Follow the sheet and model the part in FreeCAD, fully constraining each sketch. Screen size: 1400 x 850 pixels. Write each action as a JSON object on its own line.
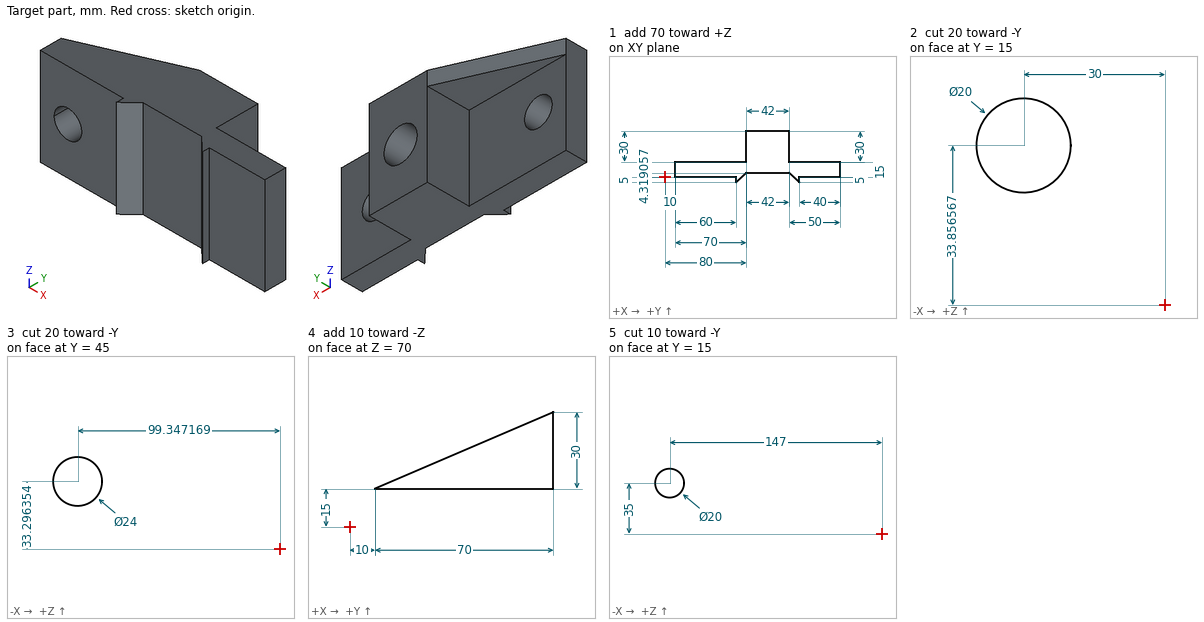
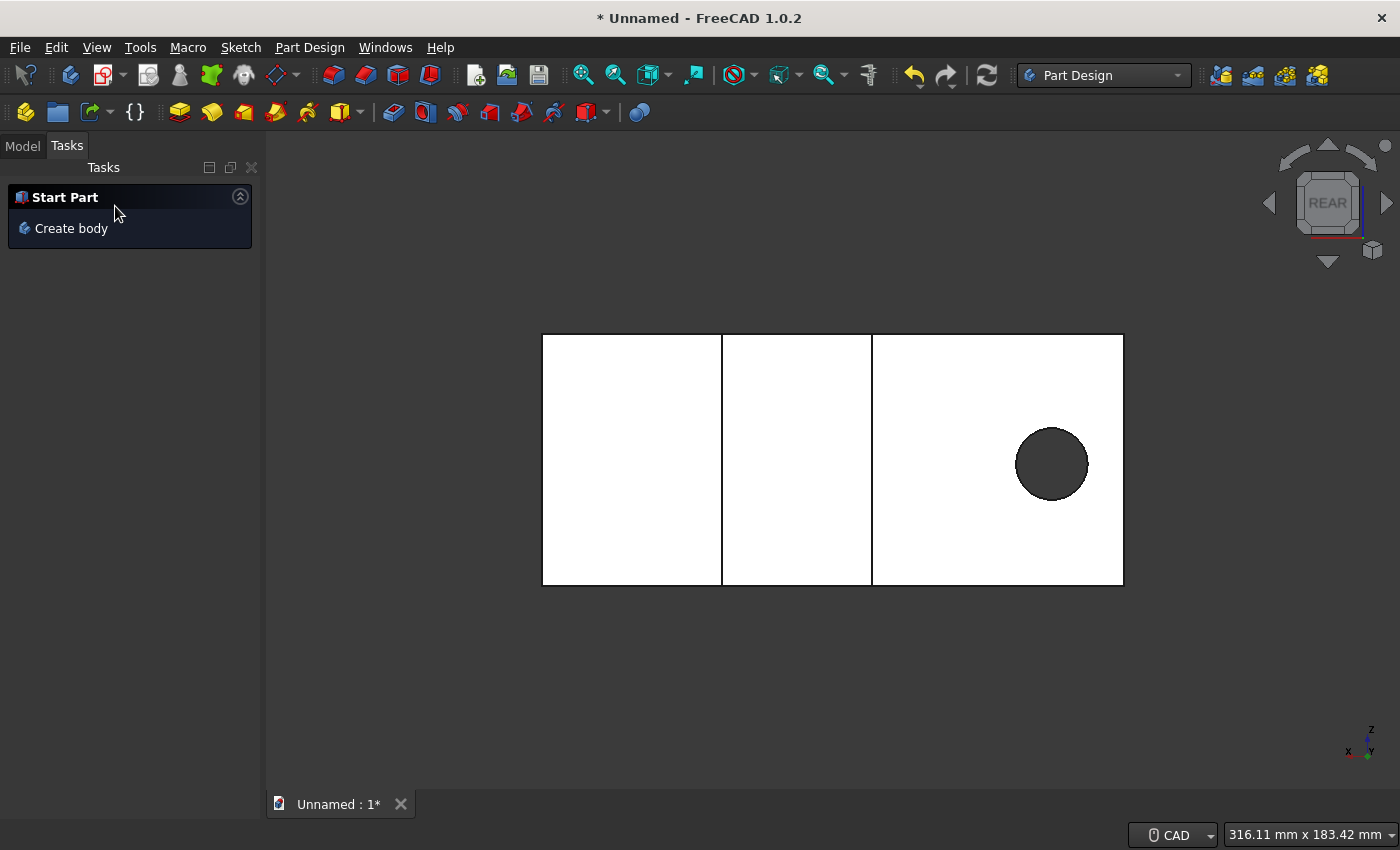
{"action": "left_click", "coordinate": [797, 423]}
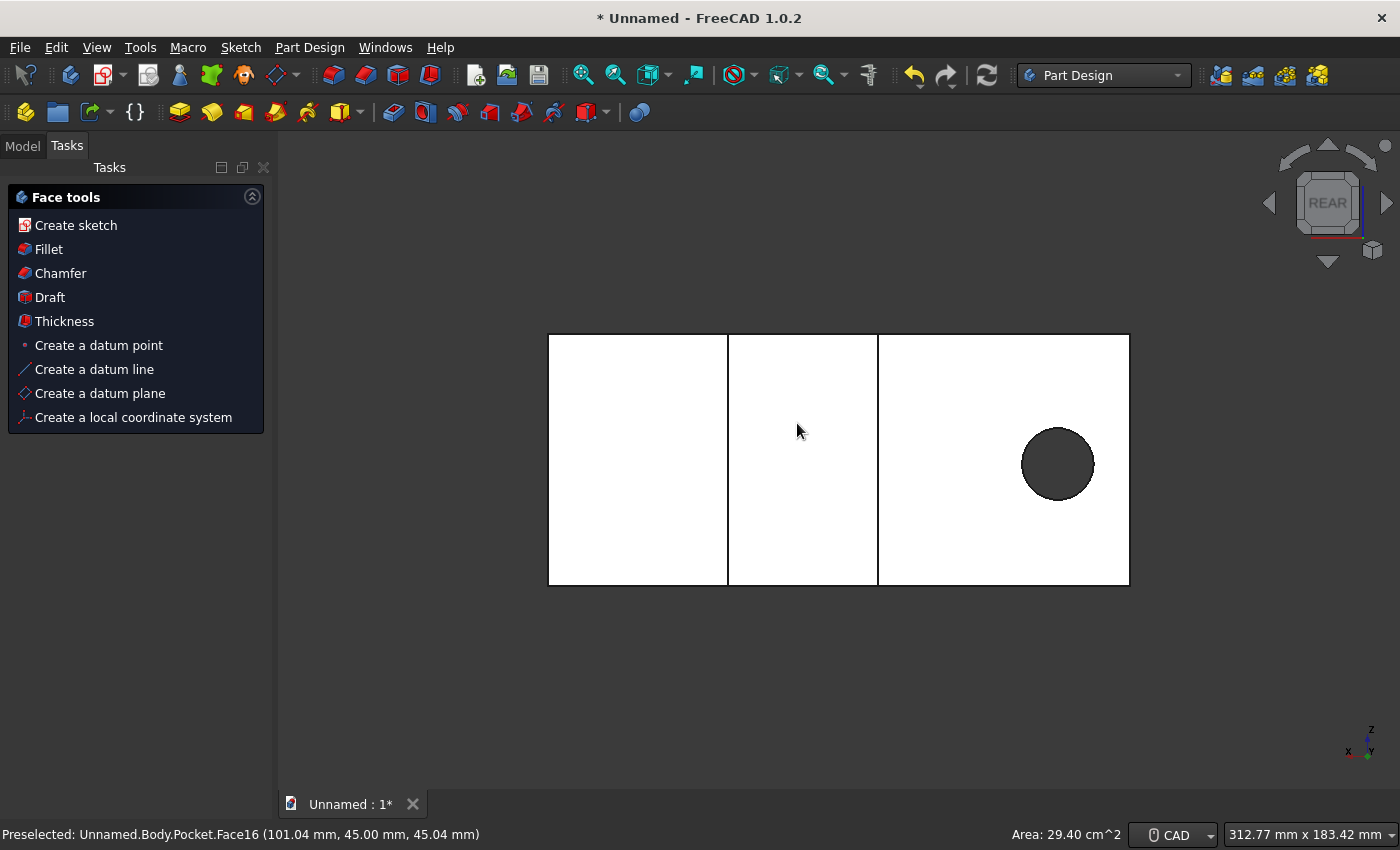
{"action": "left_click", "coordinate": [104, 76]}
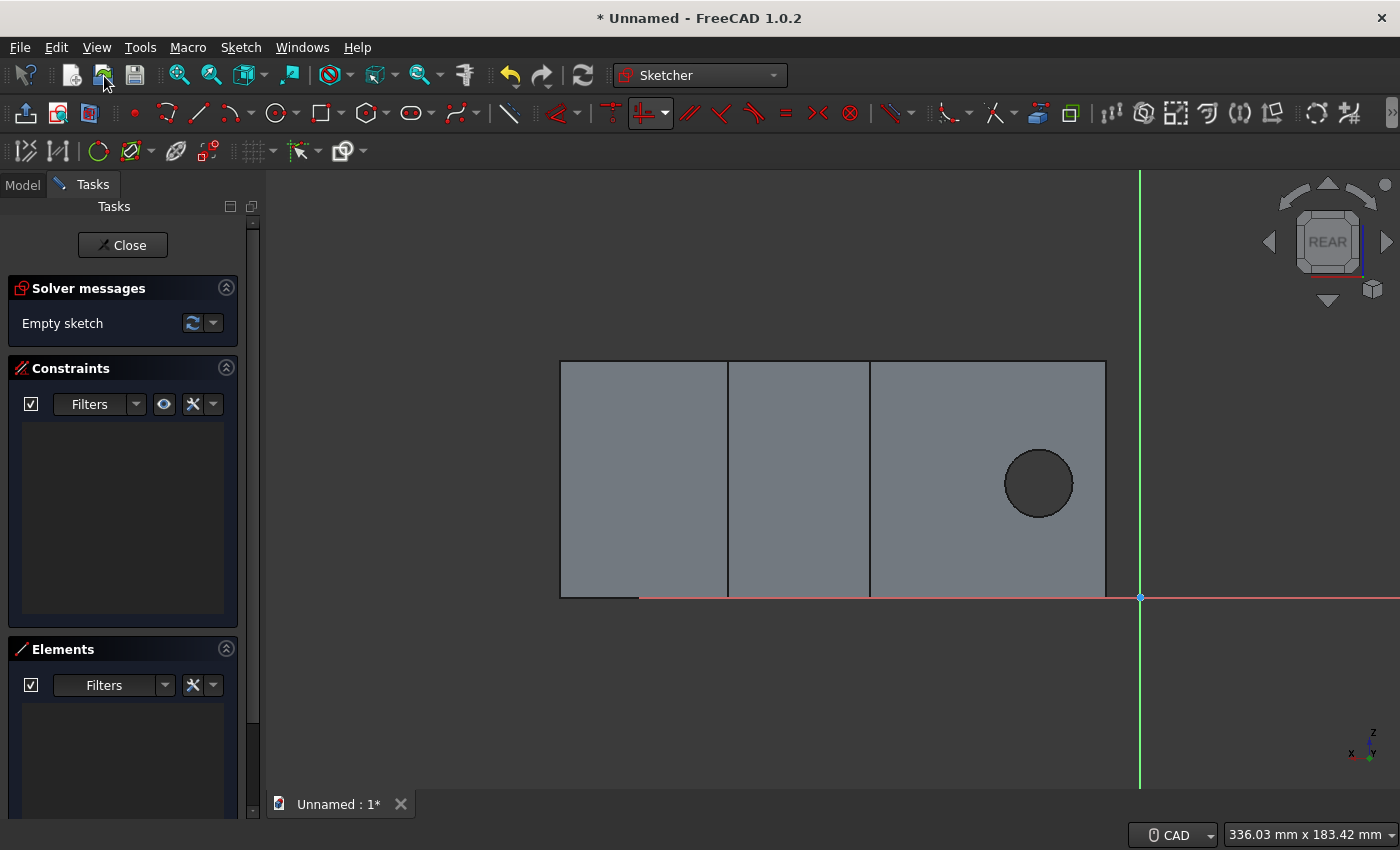
{"action": "scroll", "coordinate": [815, 487], "scroll_direction": "up", "scroll_amount": 8}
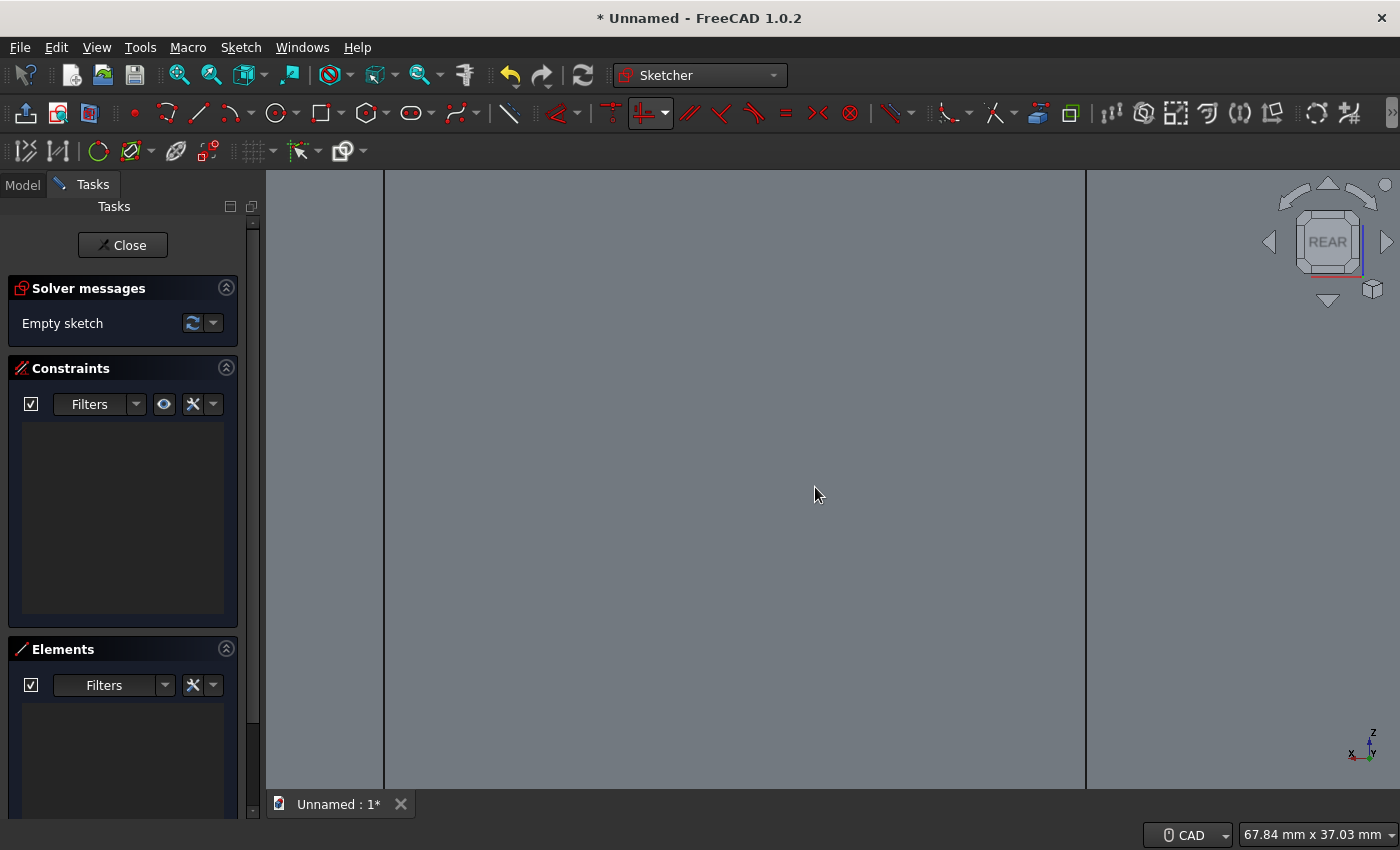
{"action": "left_click", "coordinate": [276, 114]}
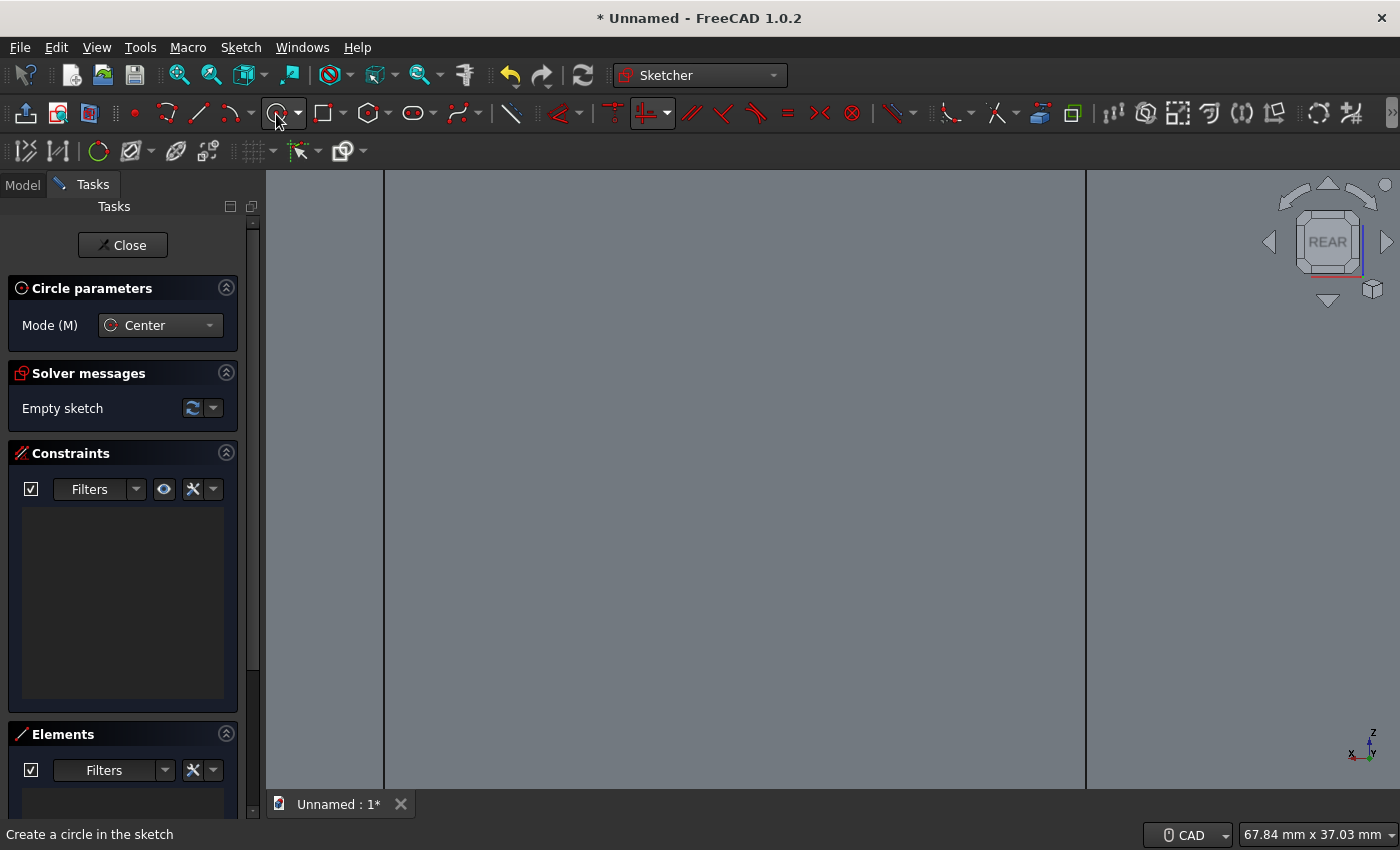
{"action": "left_click", "coordinate": [763, 476]}
{"action": "mouse_move", "coordinate": [905, 334]}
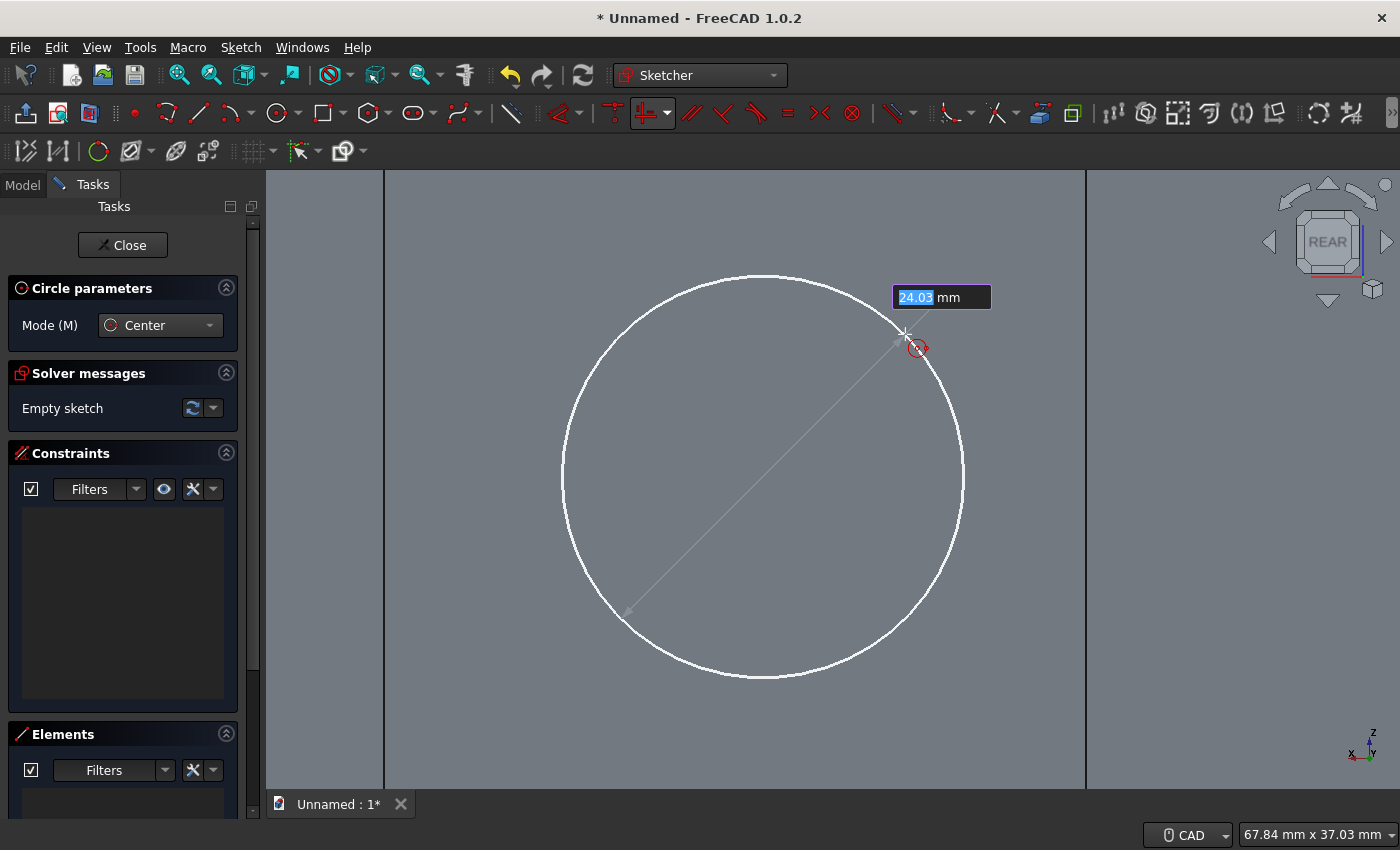
{"action": "type", "text": "24"}
{"action": "key", "text": "Return"}
{"action": "key", "text": "Escape"}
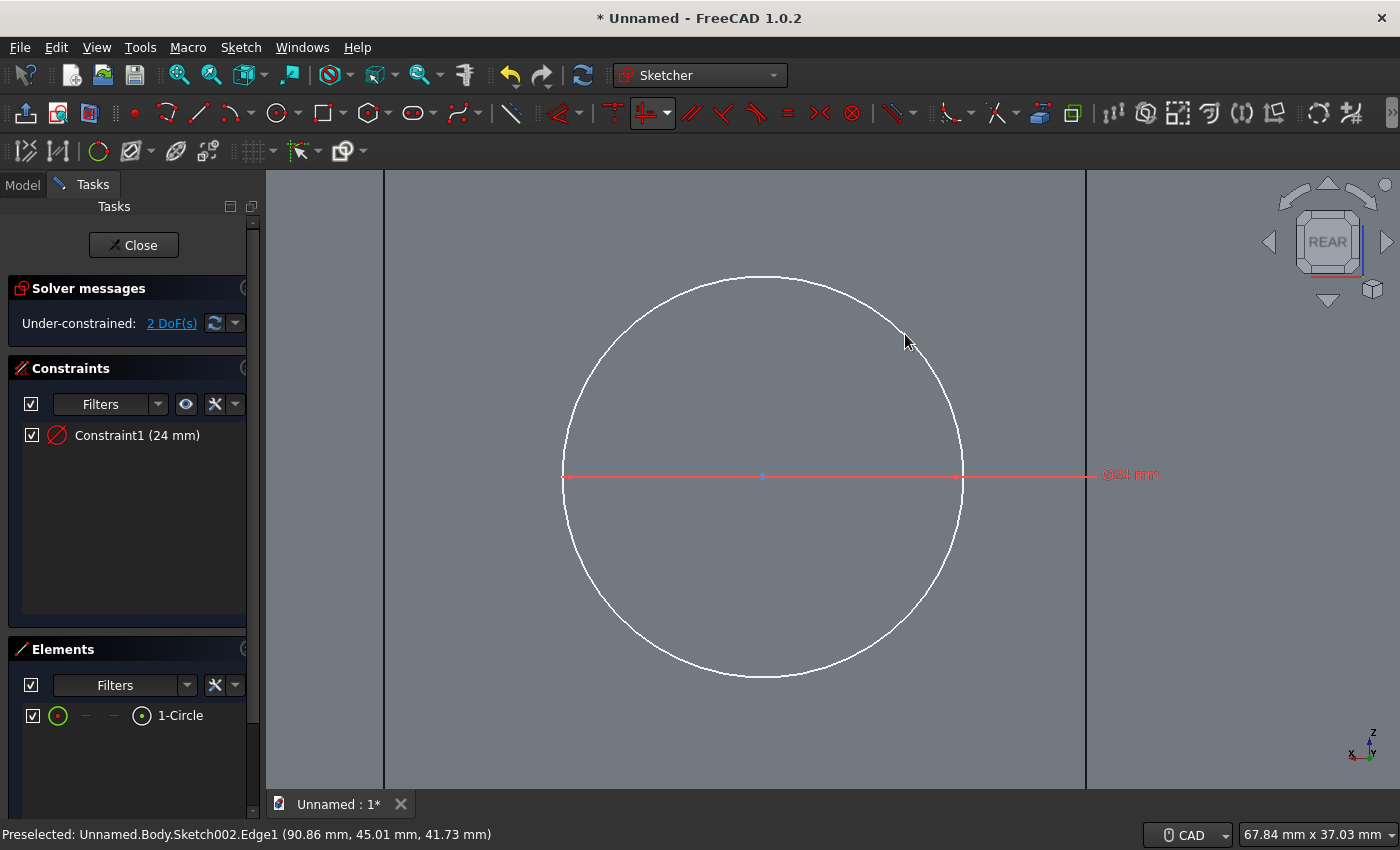
{"action": "left_click", "coordinate": [558, 114]}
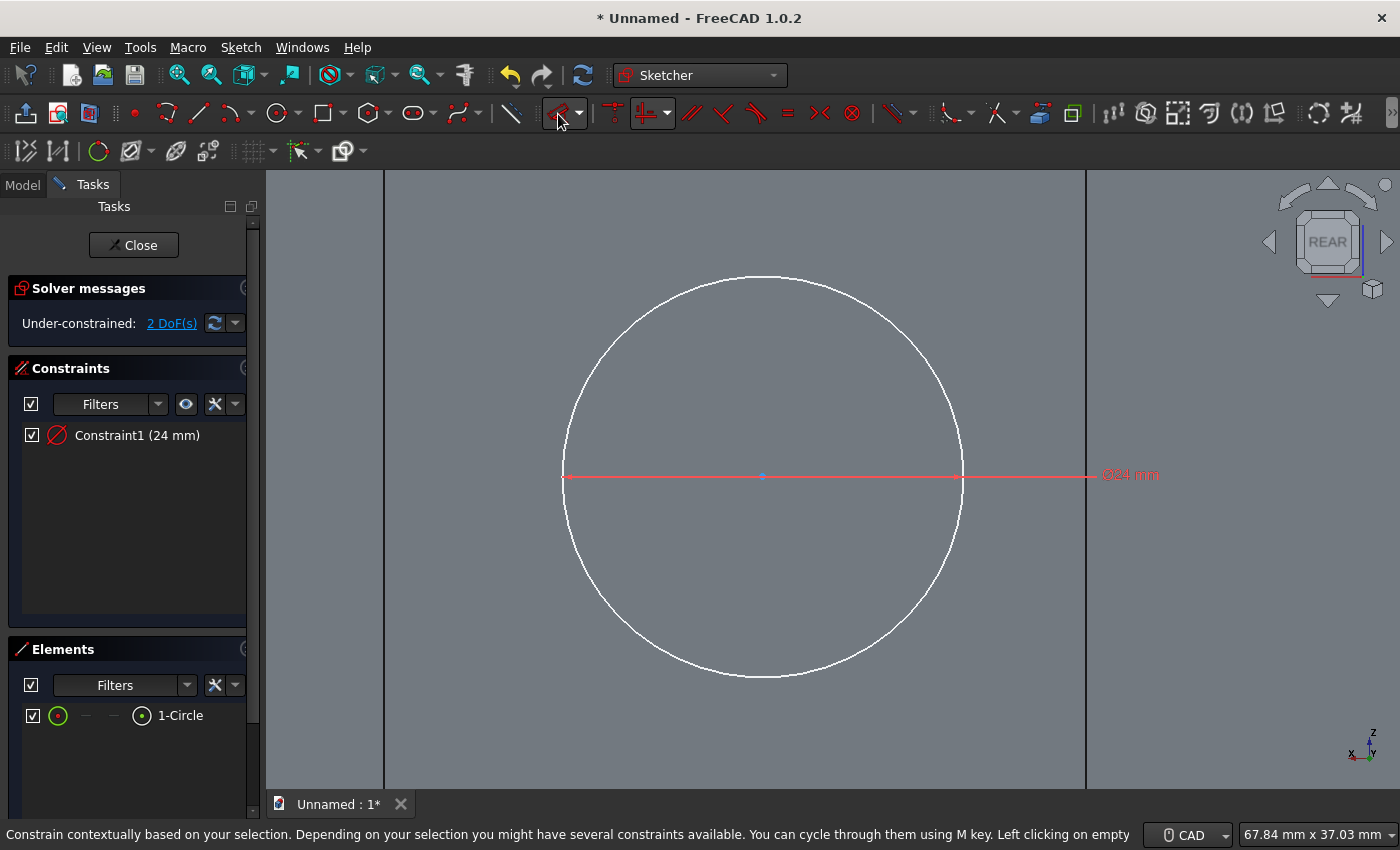
{"action": "left_click", "coordinate": [763, 477]}
{"action": "left_click", "coordinate": [999, 443]}